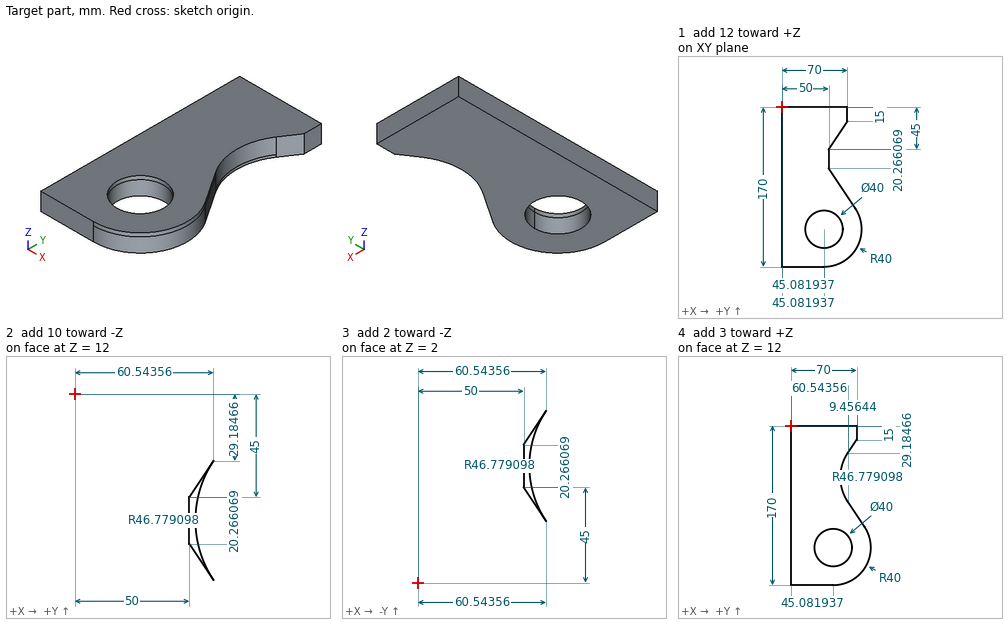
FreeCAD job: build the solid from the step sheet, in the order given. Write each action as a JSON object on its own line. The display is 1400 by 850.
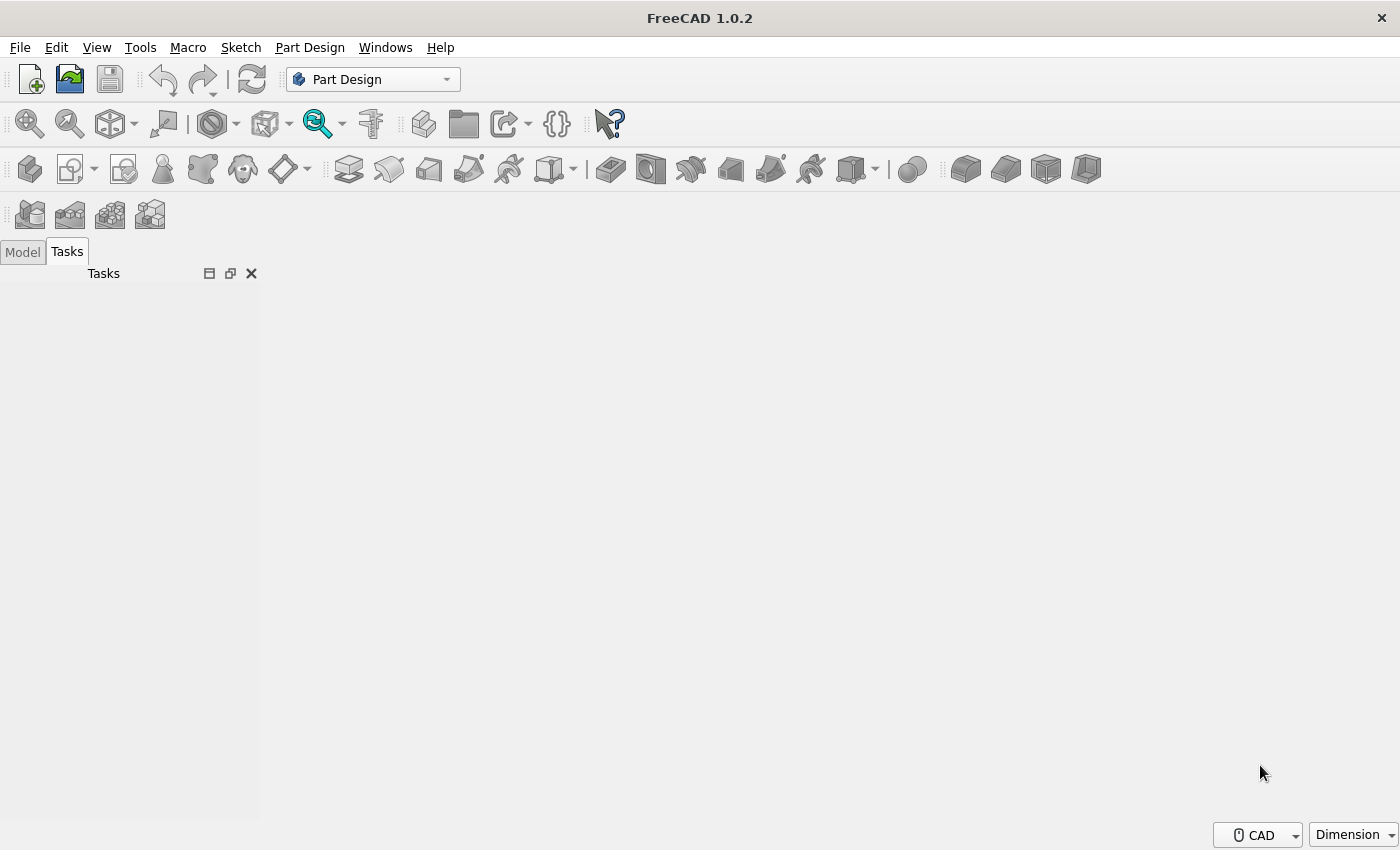
{"action": "left_click", "coordinate": [30, 80]}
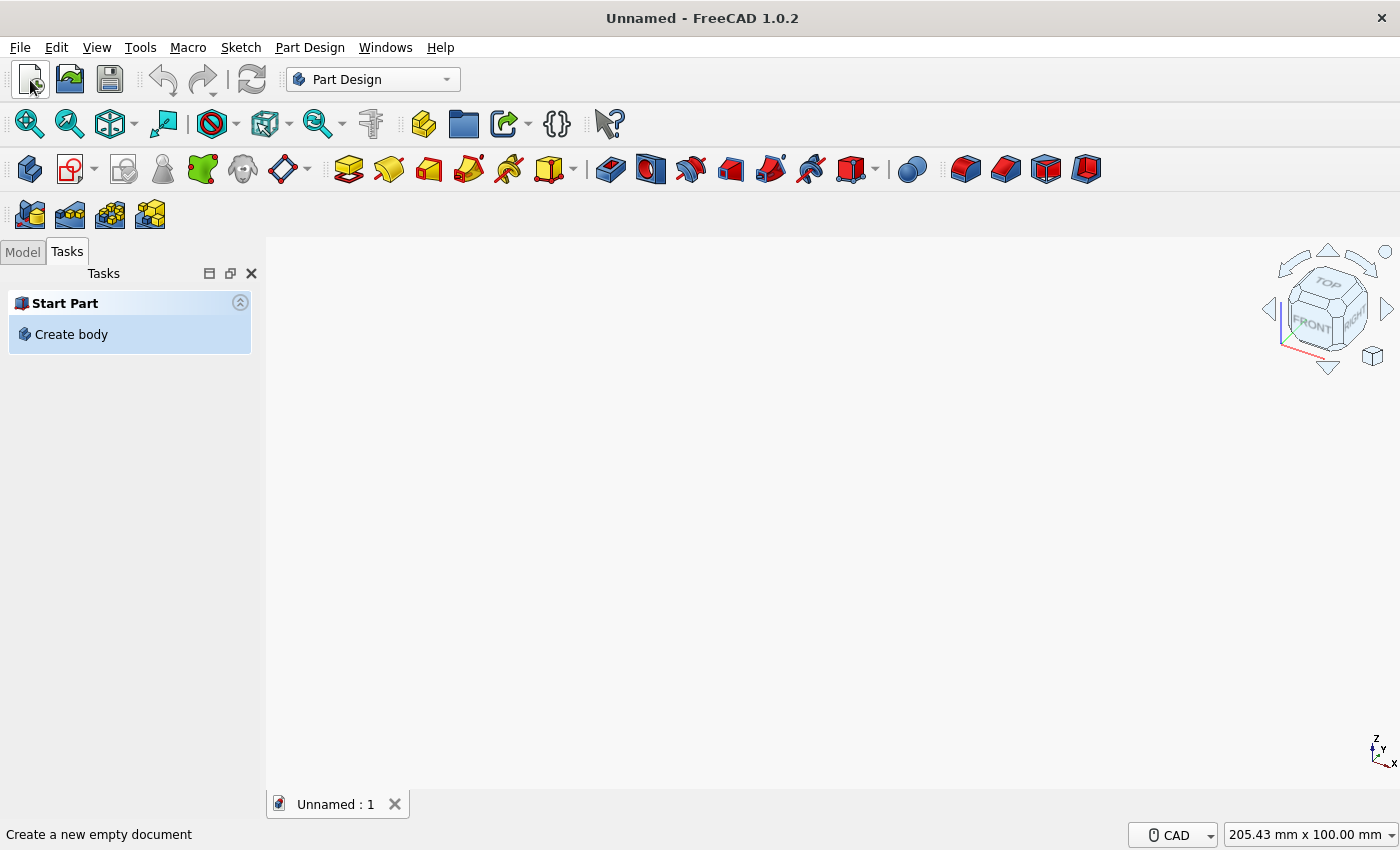
{"action": "left_click", "coordinate": [70, 170]}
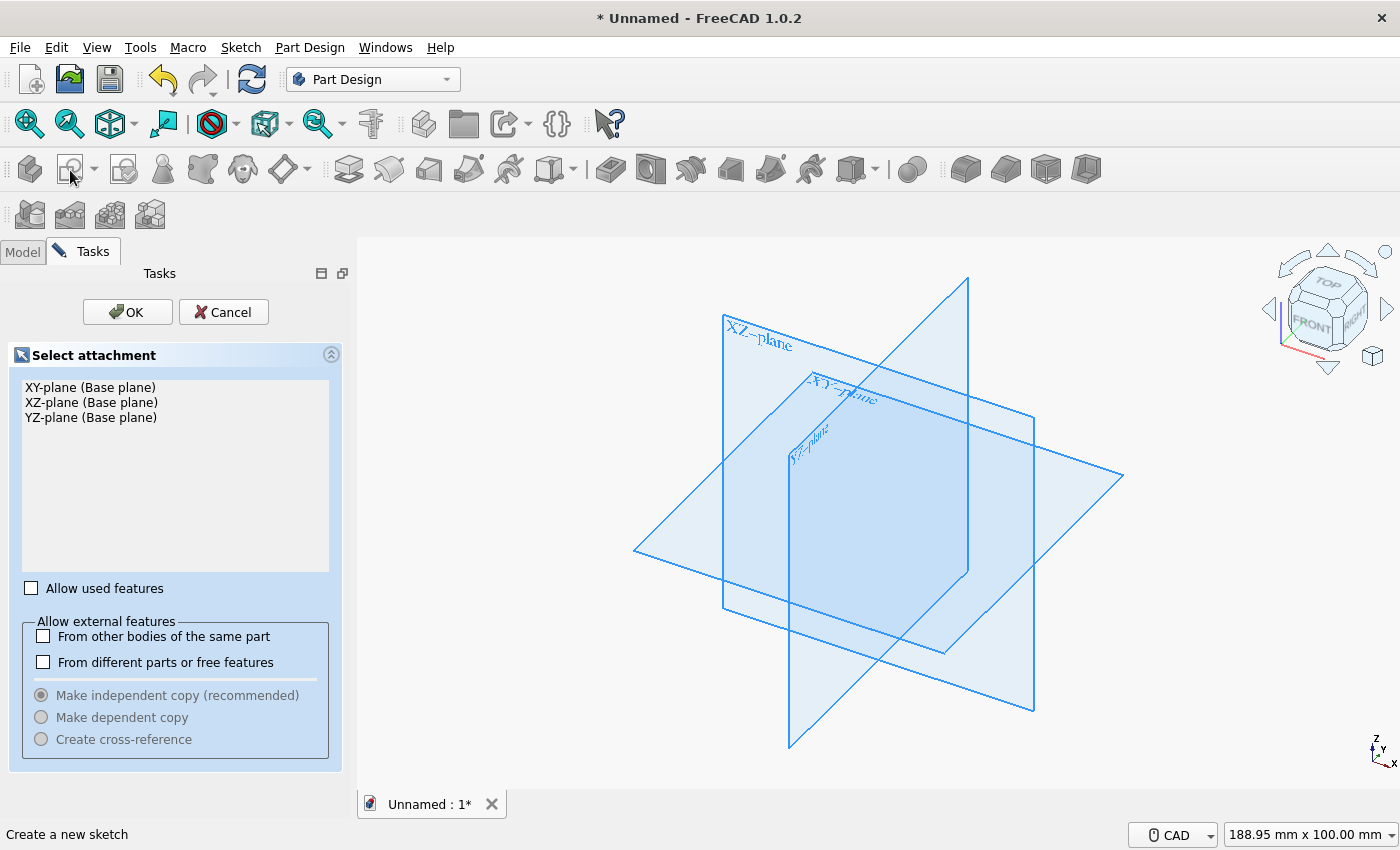
{"action": "left_click", "coordinate": [82, 388]}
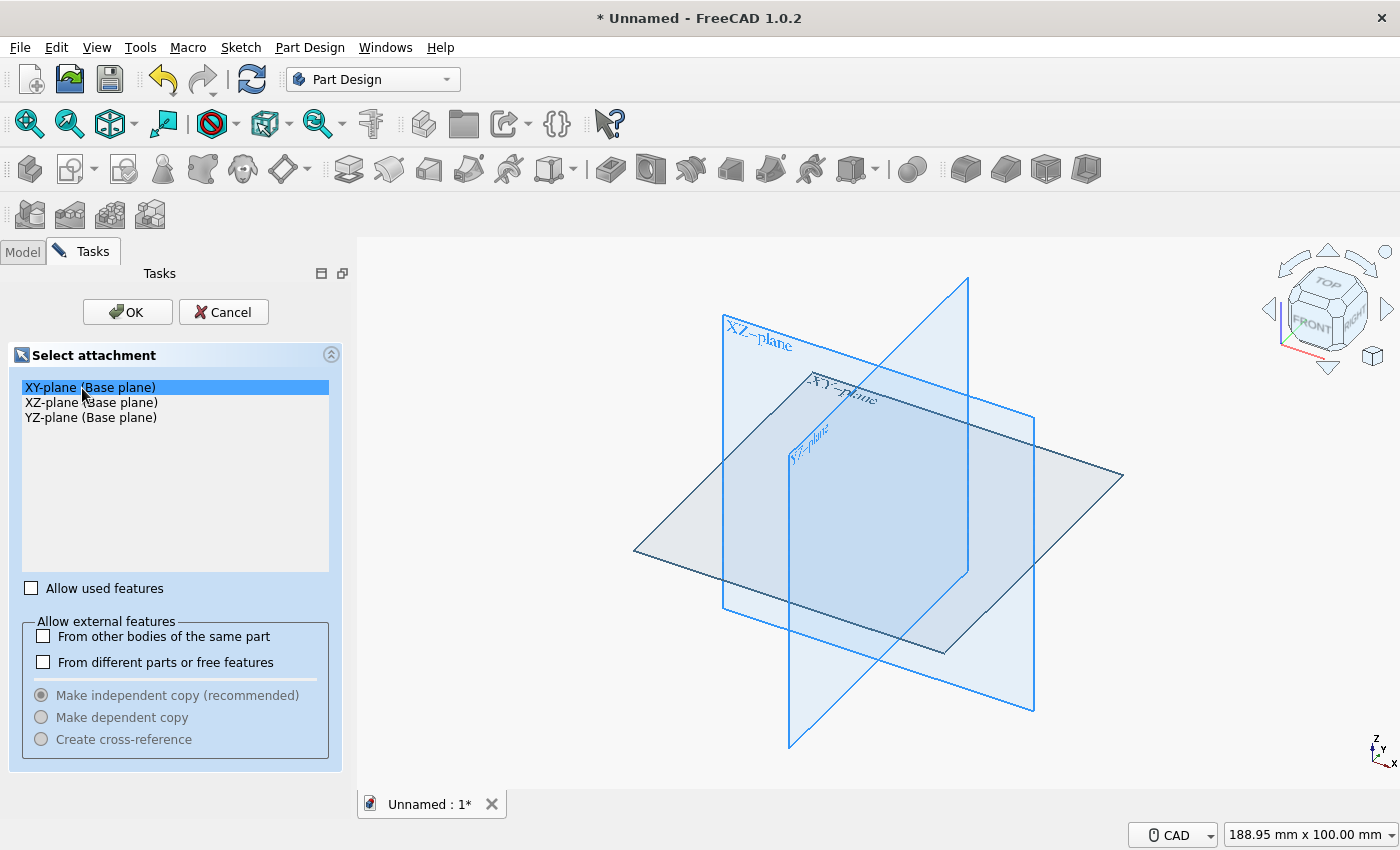
{"action": "left_click", "coordinate": [128, 312]}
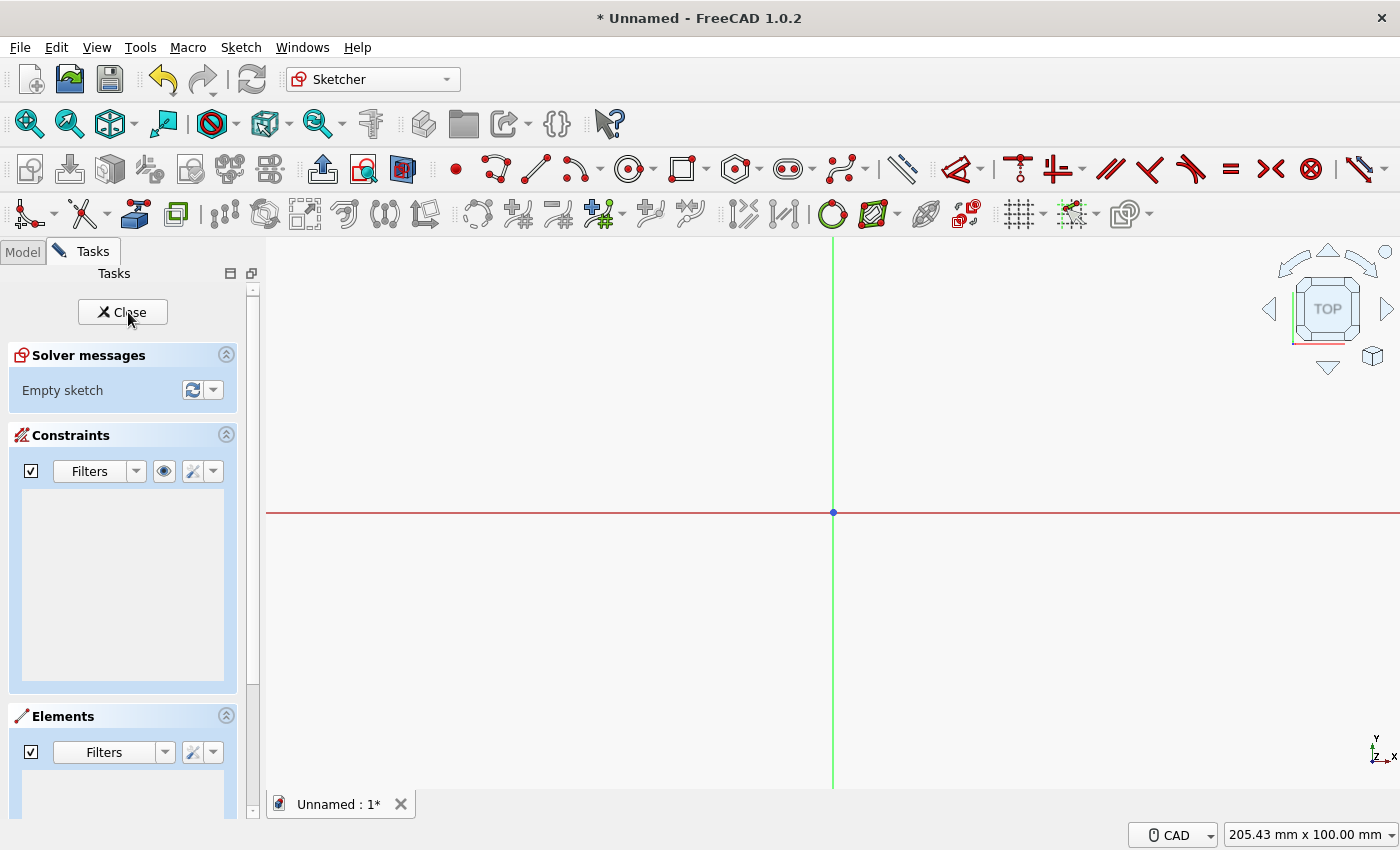
{"action": "scroll", "coordinate": [596, 265], "scroll_direction": "down", "scroll_amount": 5}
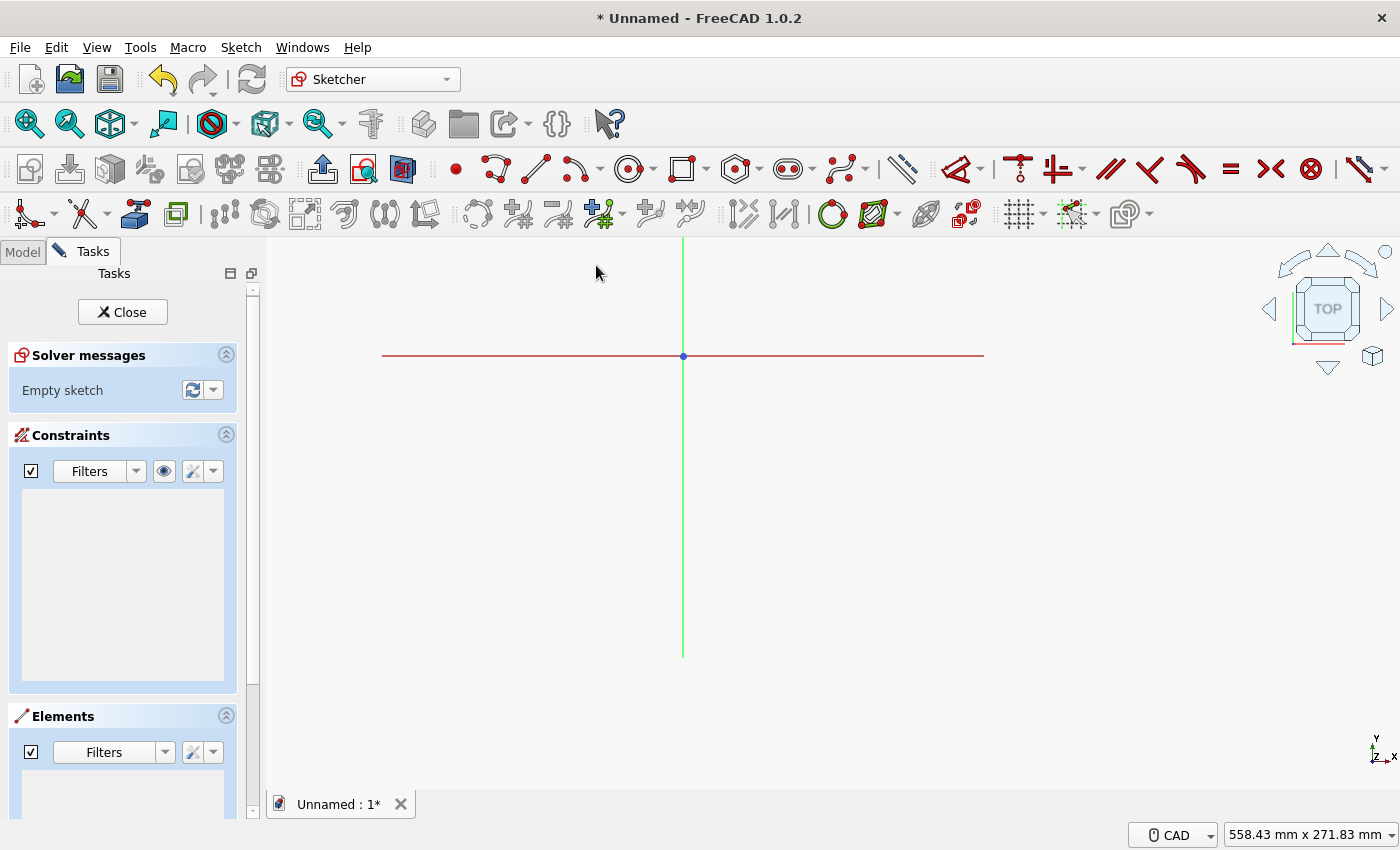
{"action": "left_click", "coordinate": [496, 170]}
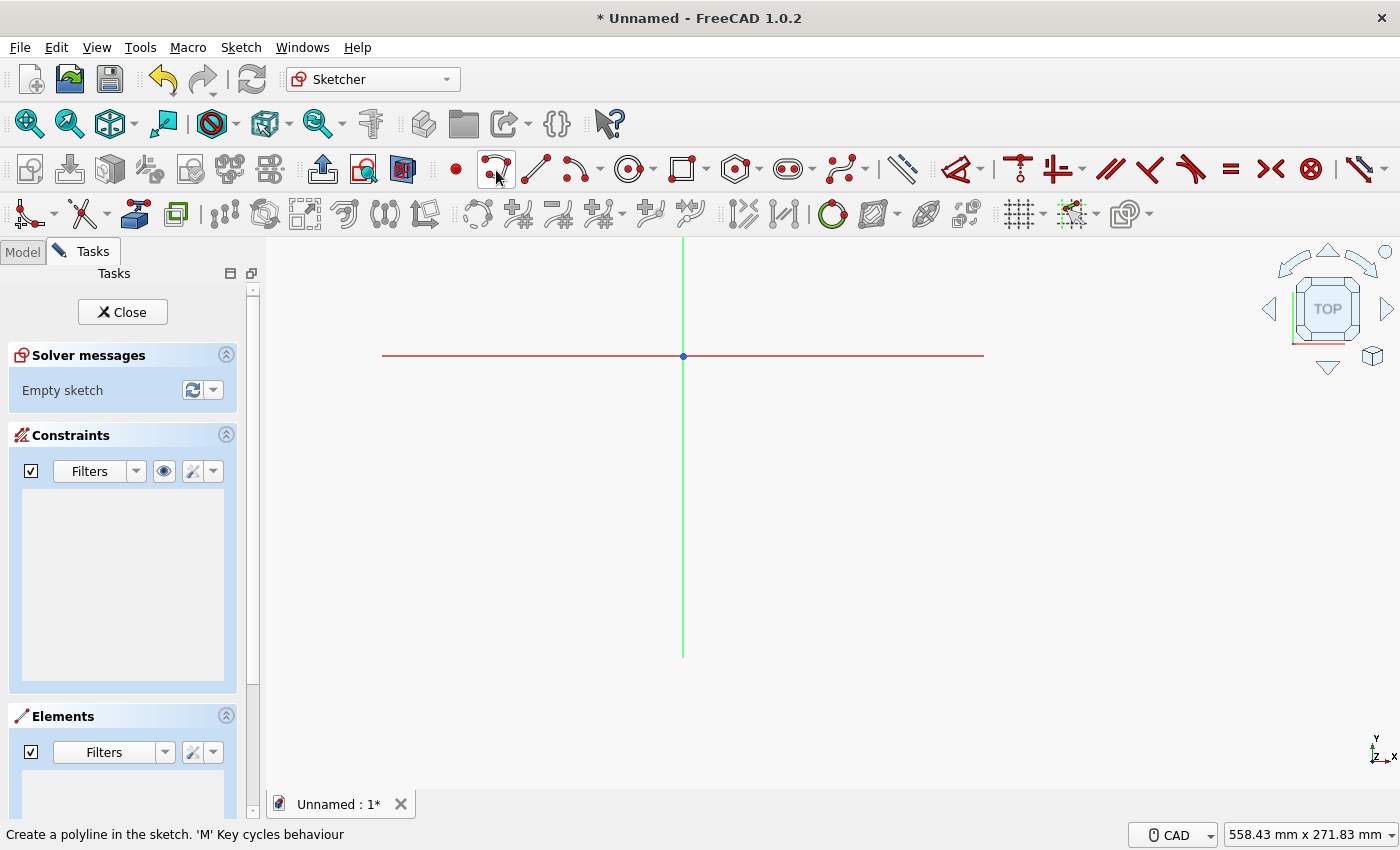
{"action": "left_click", "coordinate": [843, 575]}
{"action": "left_click", "coordinate": [785, 489]}
{"action": "left_click", "coordinate": [785, 448]}
{"action": "left_click", "coordinate": [826, 387]}
{"action": "left_click", "coordinate": [826, 356]}
{"action": "left_click", "coordinate": [683, 356]}
{"action": "left_click", "coordinate": [692, 701]}
{"action": "left_click", "coordinate": [775, 701]}
{"action": "right_click", "coordinate": [775, 701]}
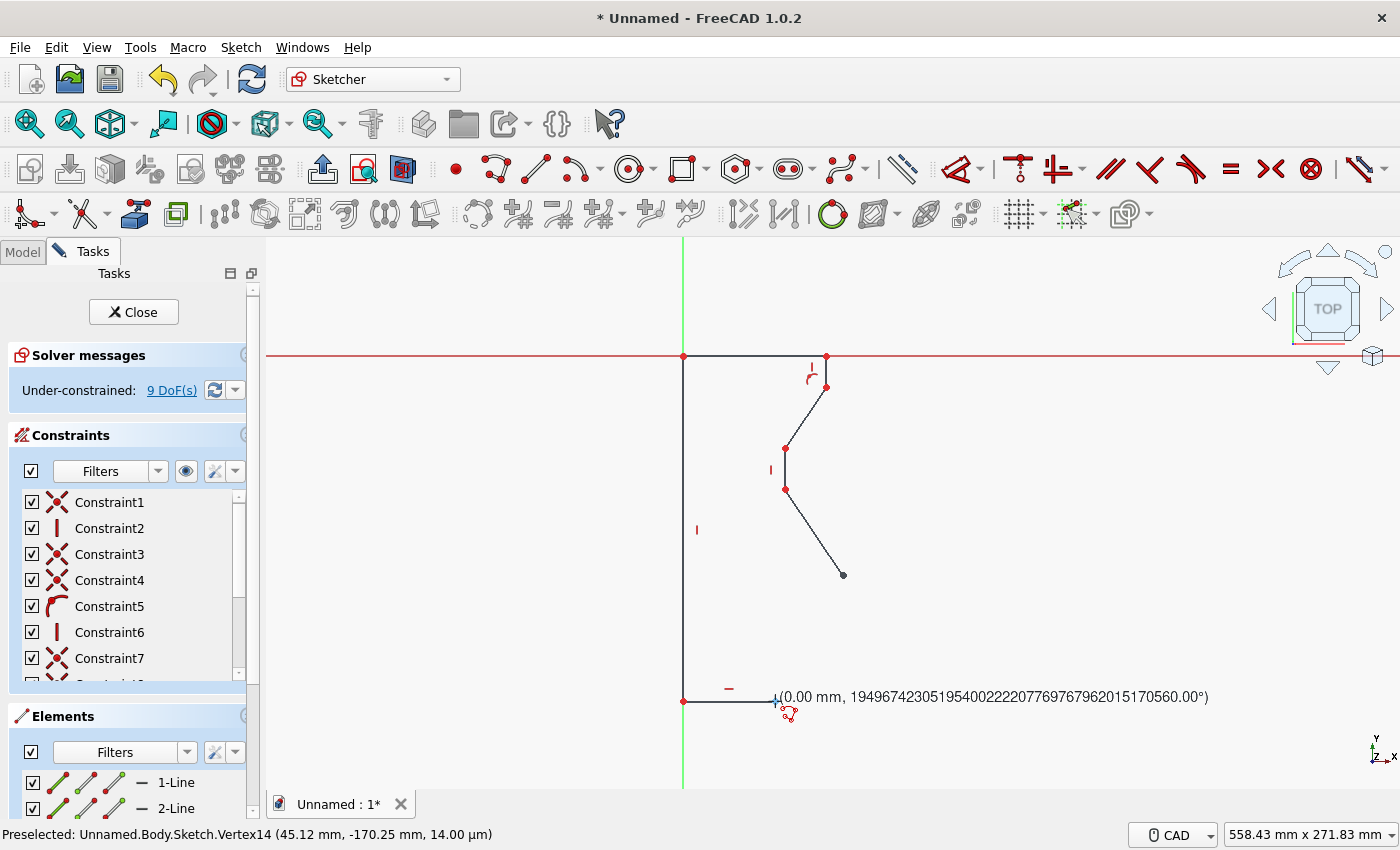
{"action": "left_click", "coordinate": [602, 170]}